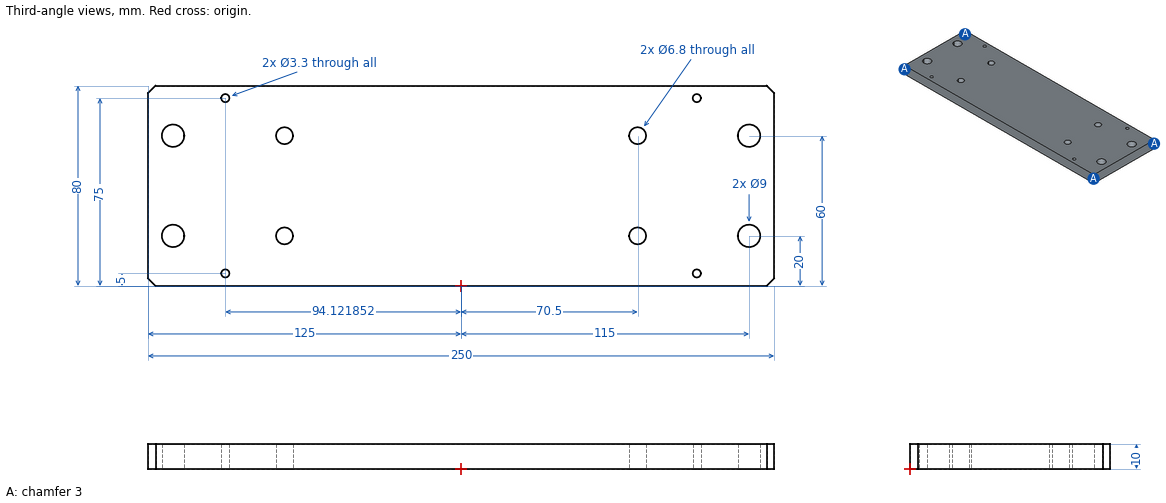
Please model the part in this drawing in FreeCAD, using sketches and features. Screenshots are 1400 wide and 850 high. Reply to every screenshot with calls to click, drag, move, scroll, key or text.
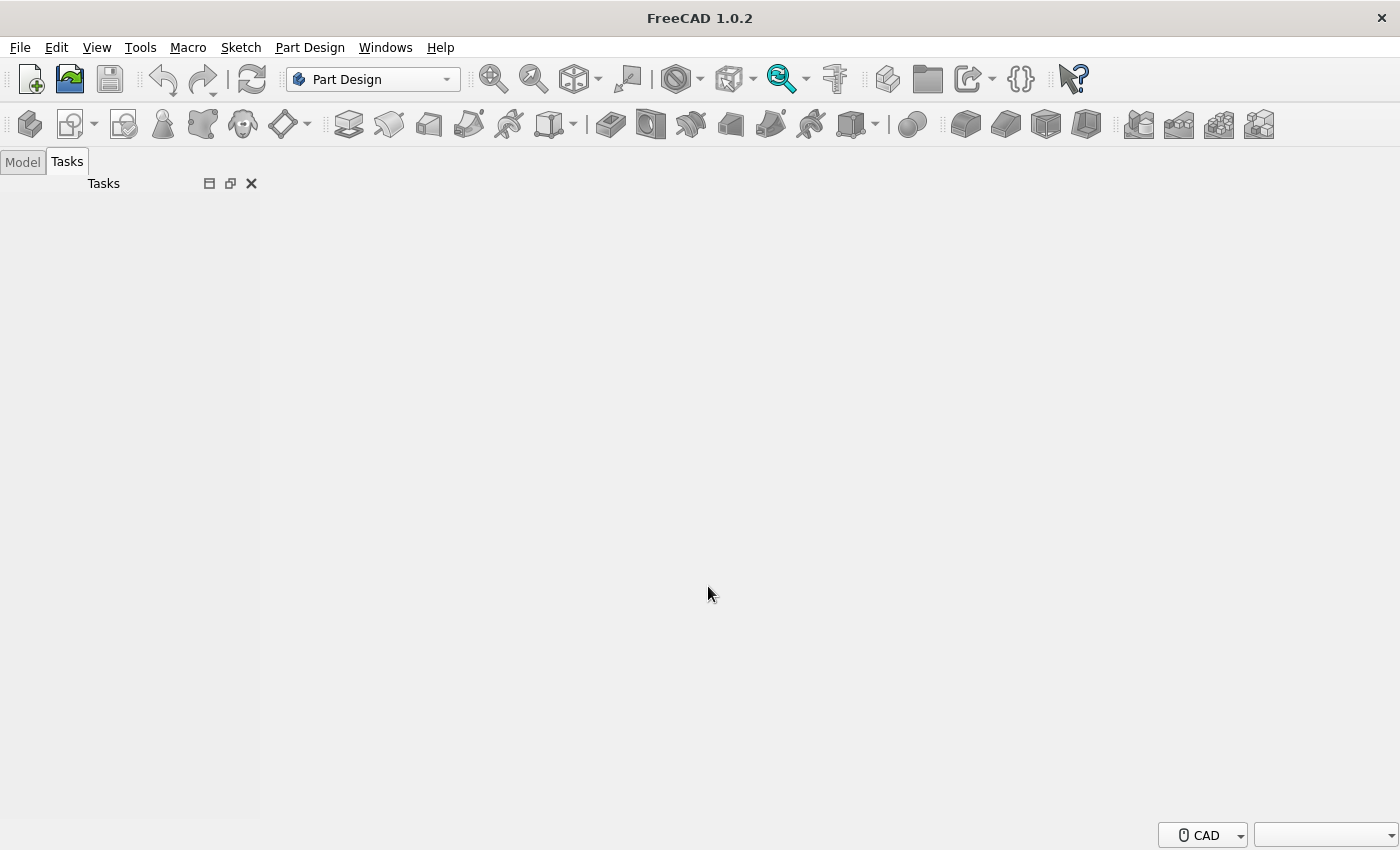
click(30, 80)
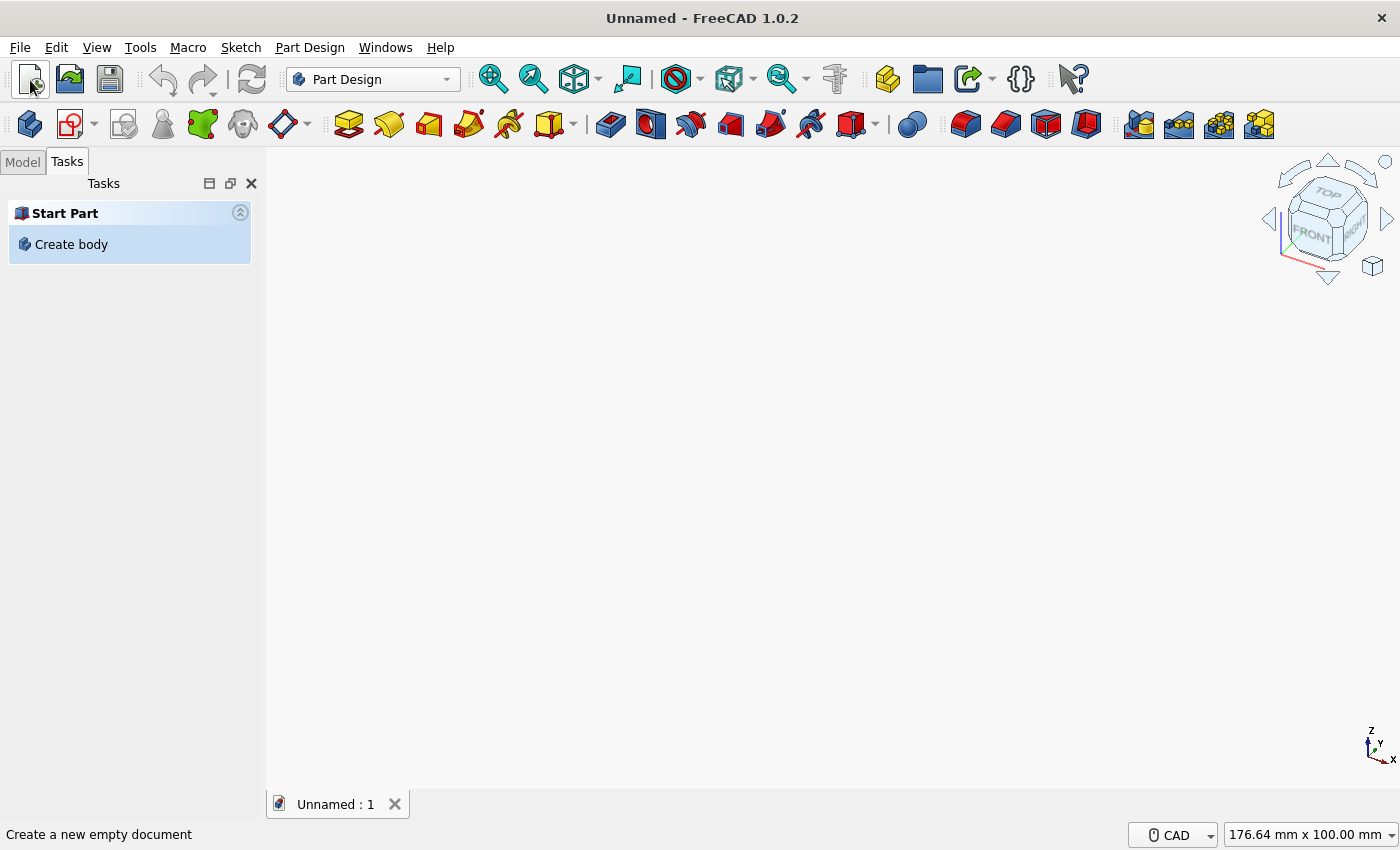
click(70, 124)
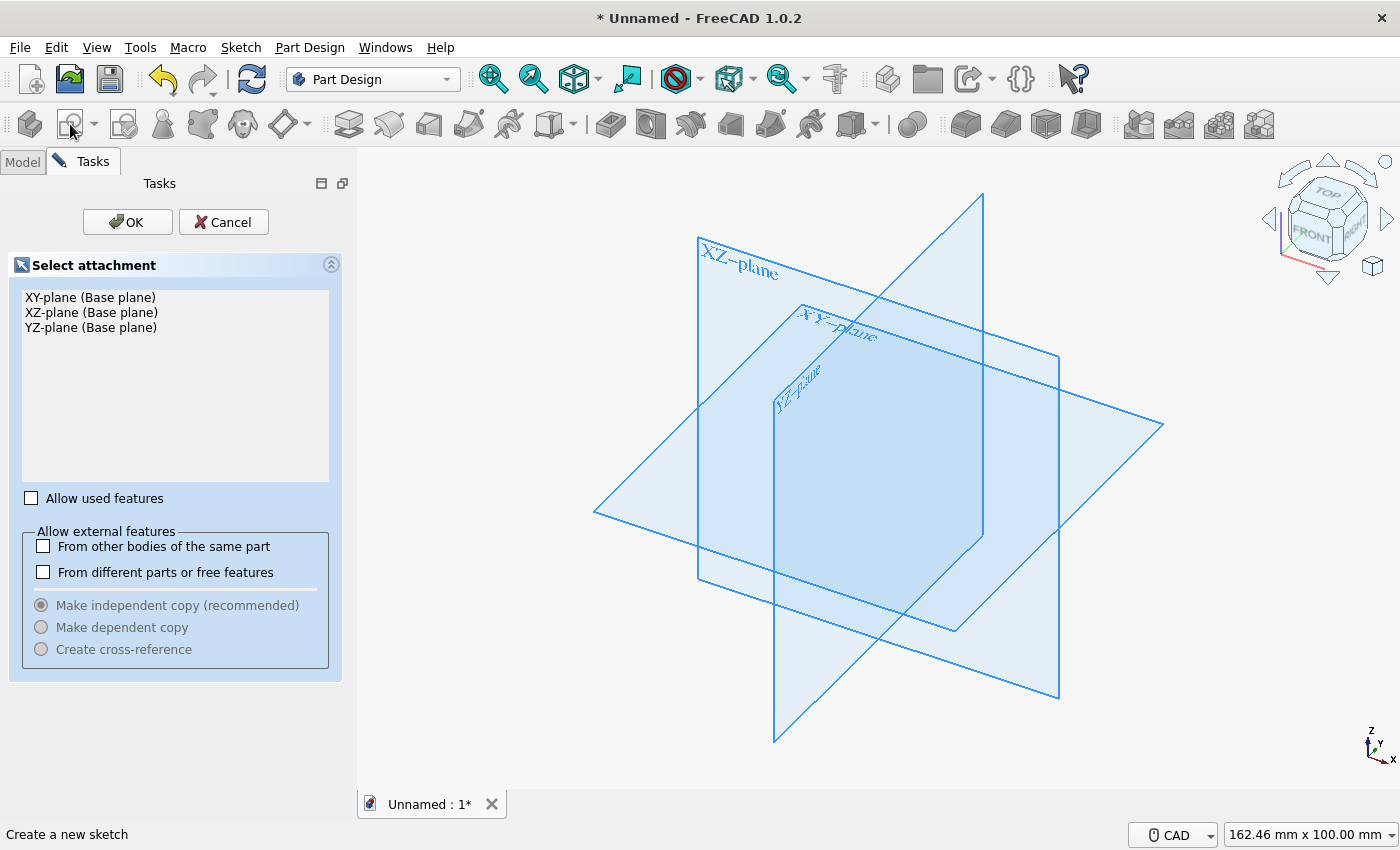
click(82, 298)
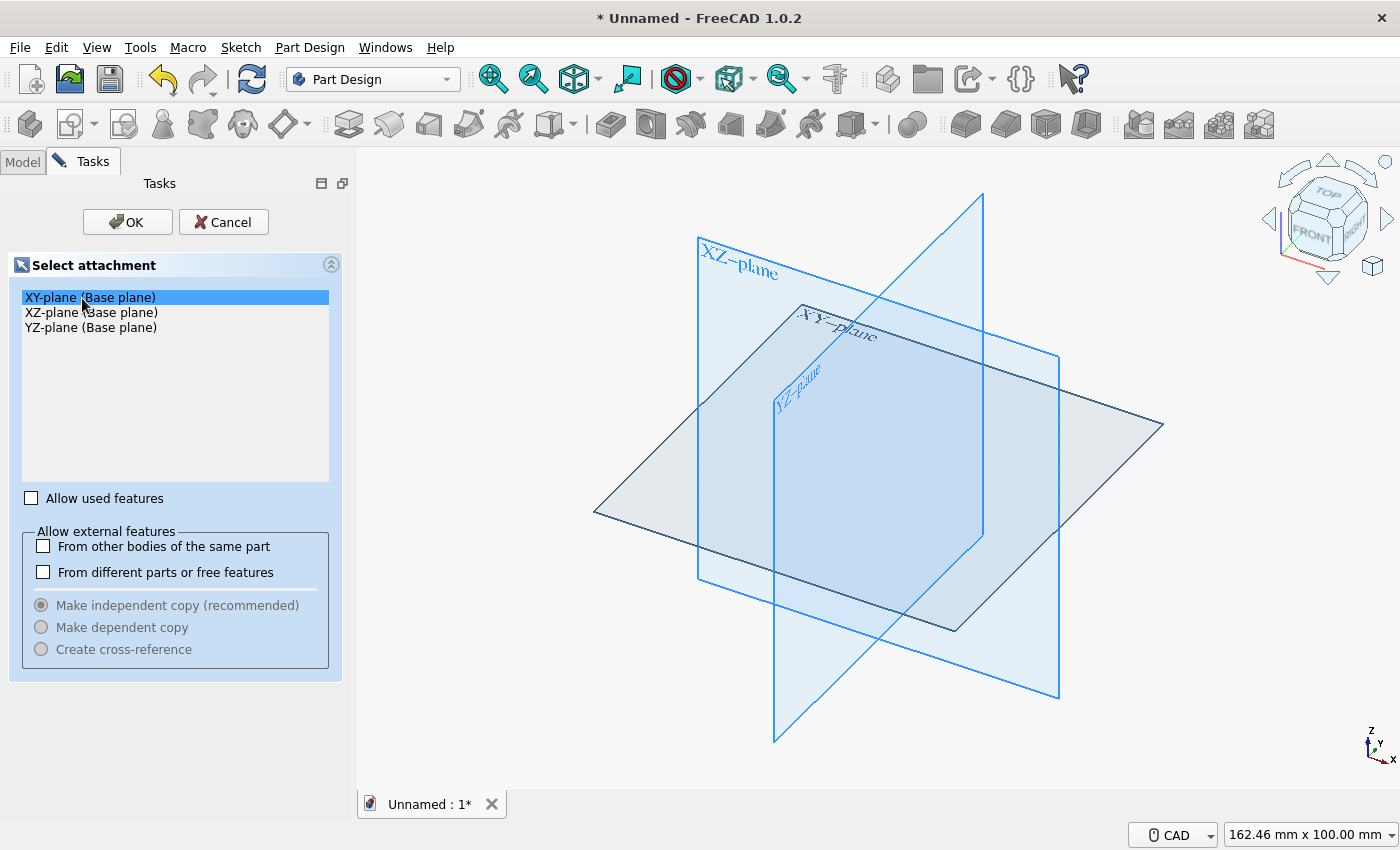
click(128, 222)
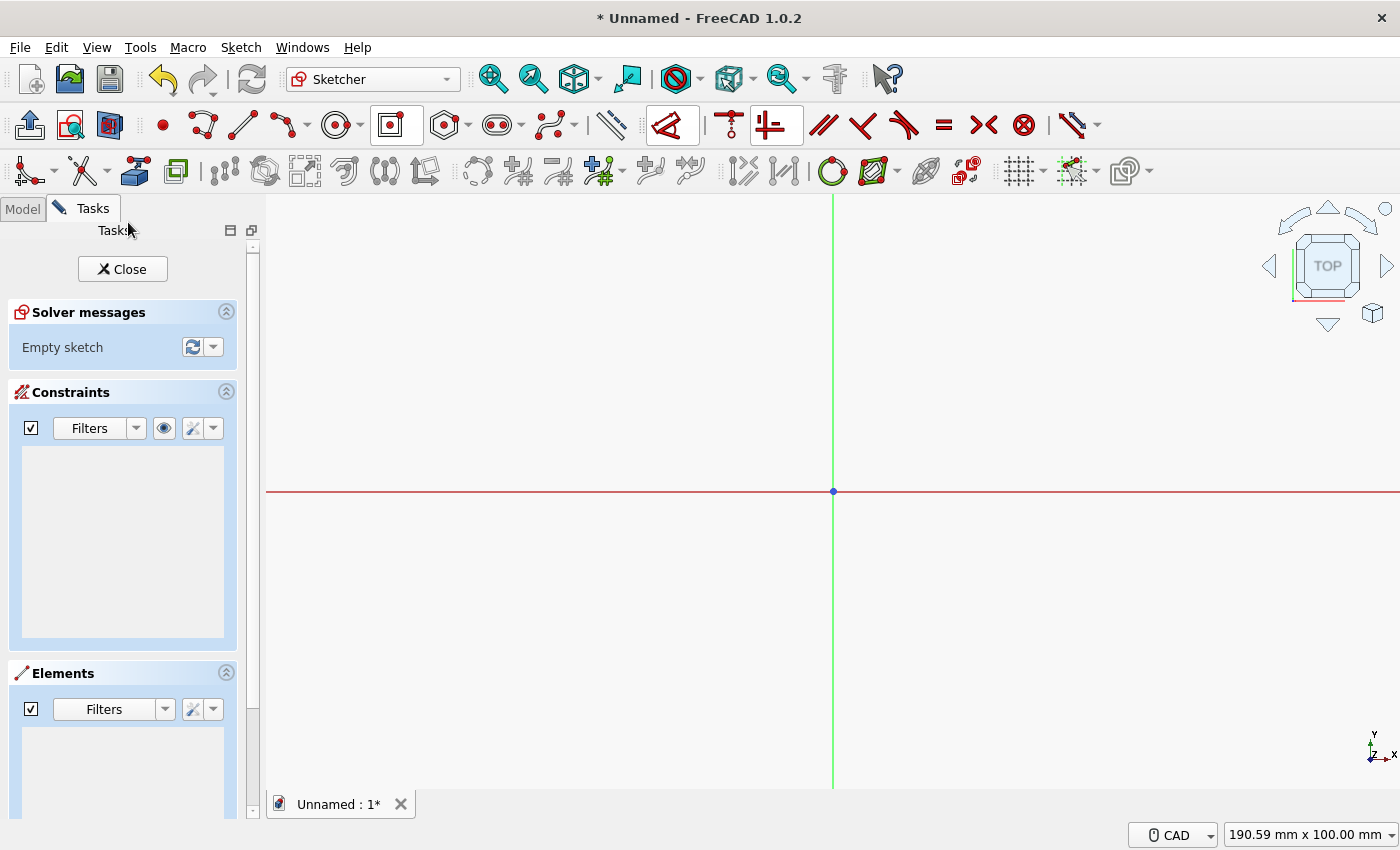
scroll(709, 686, down, 4)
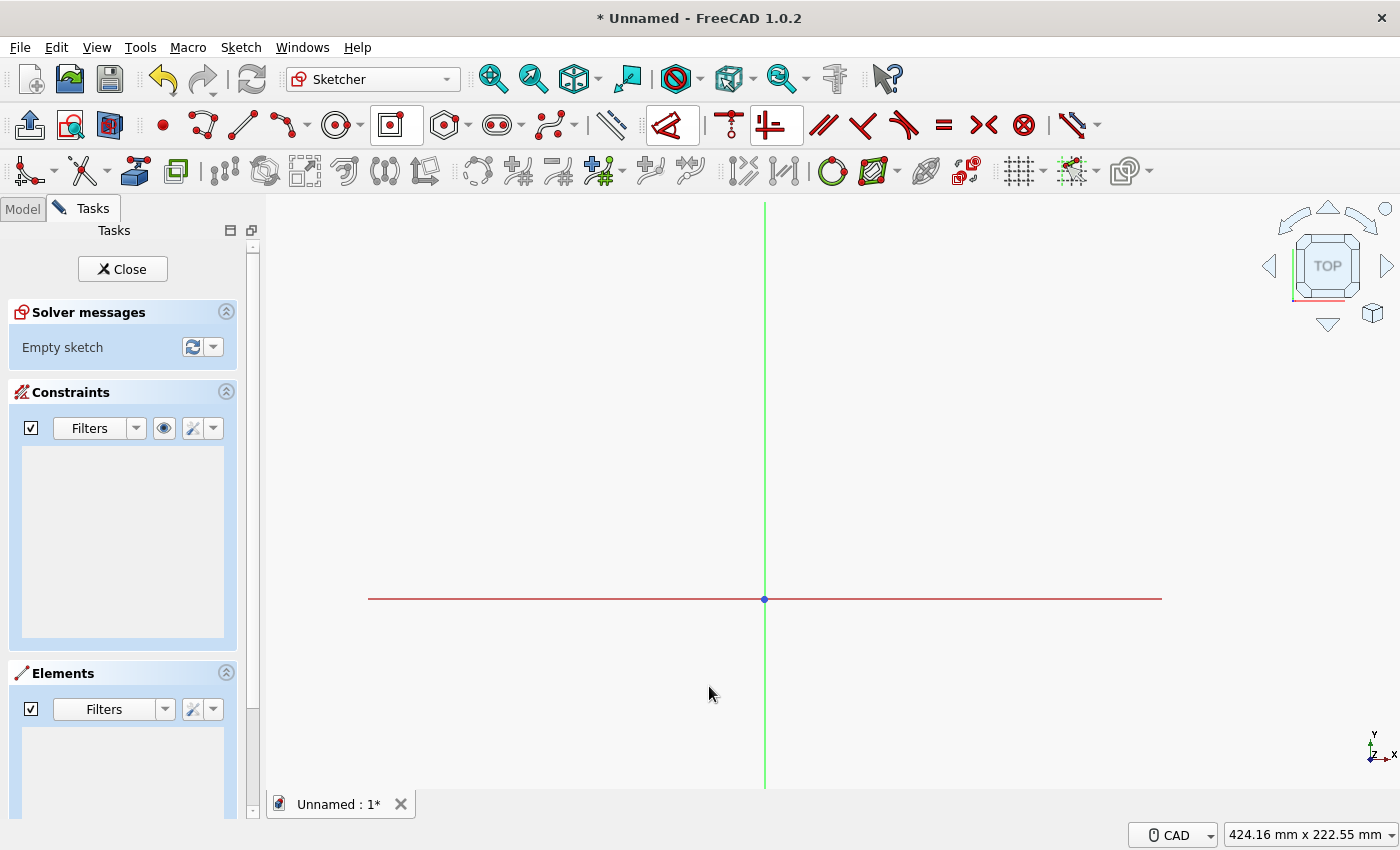
key(g)
key(r)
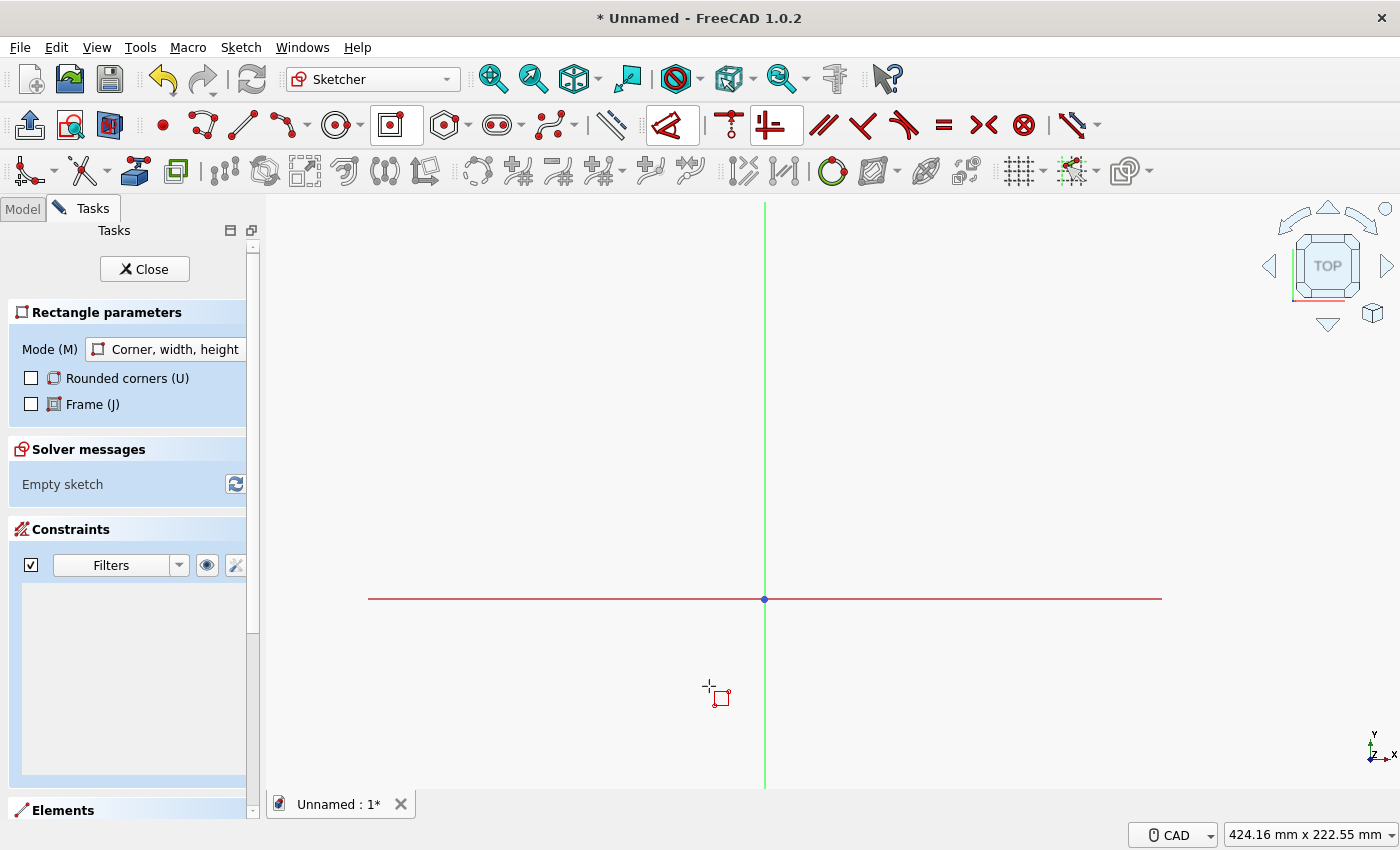
click(431, 385)
click(1099, 599)
key(Escape)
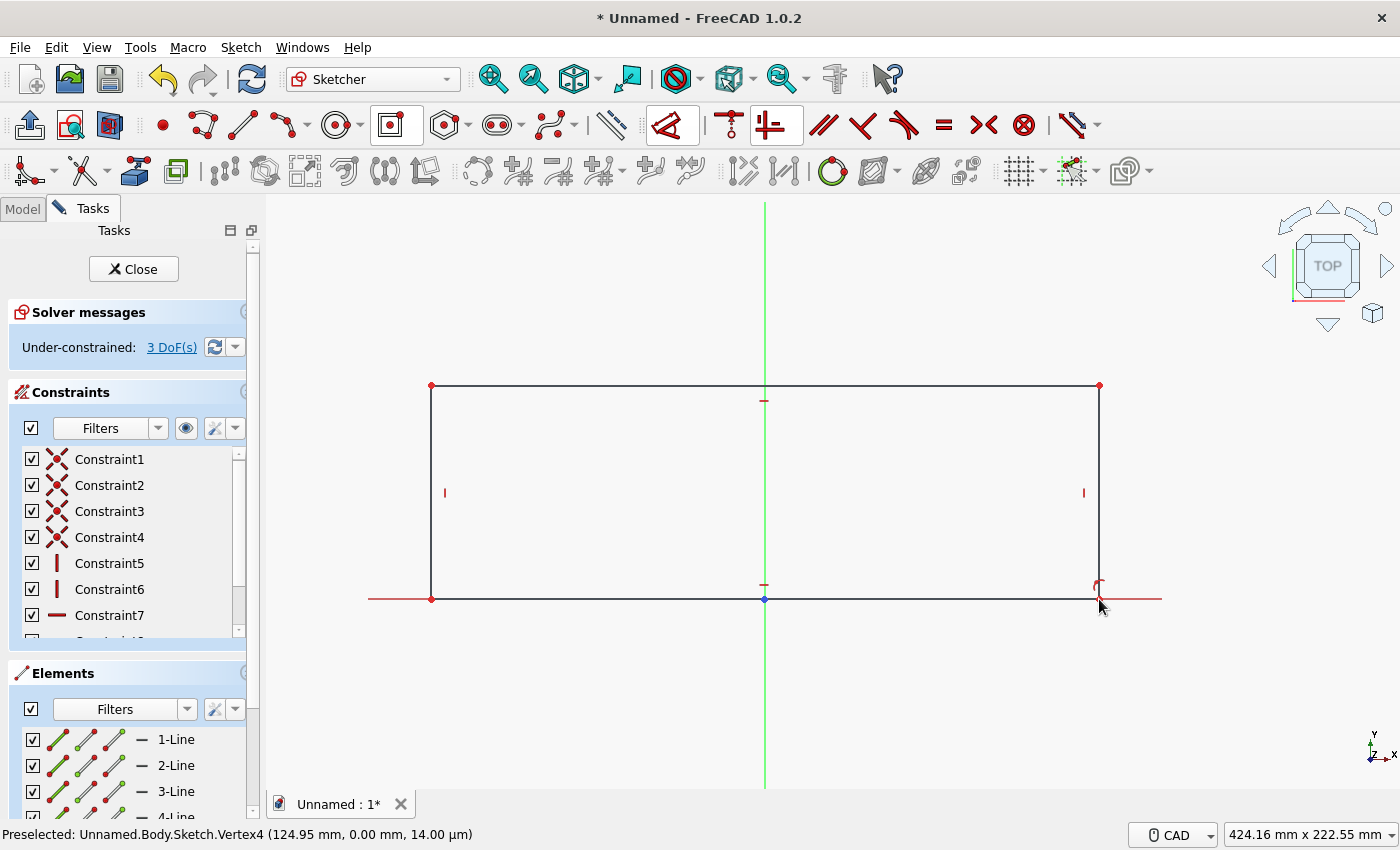
click(666, 126)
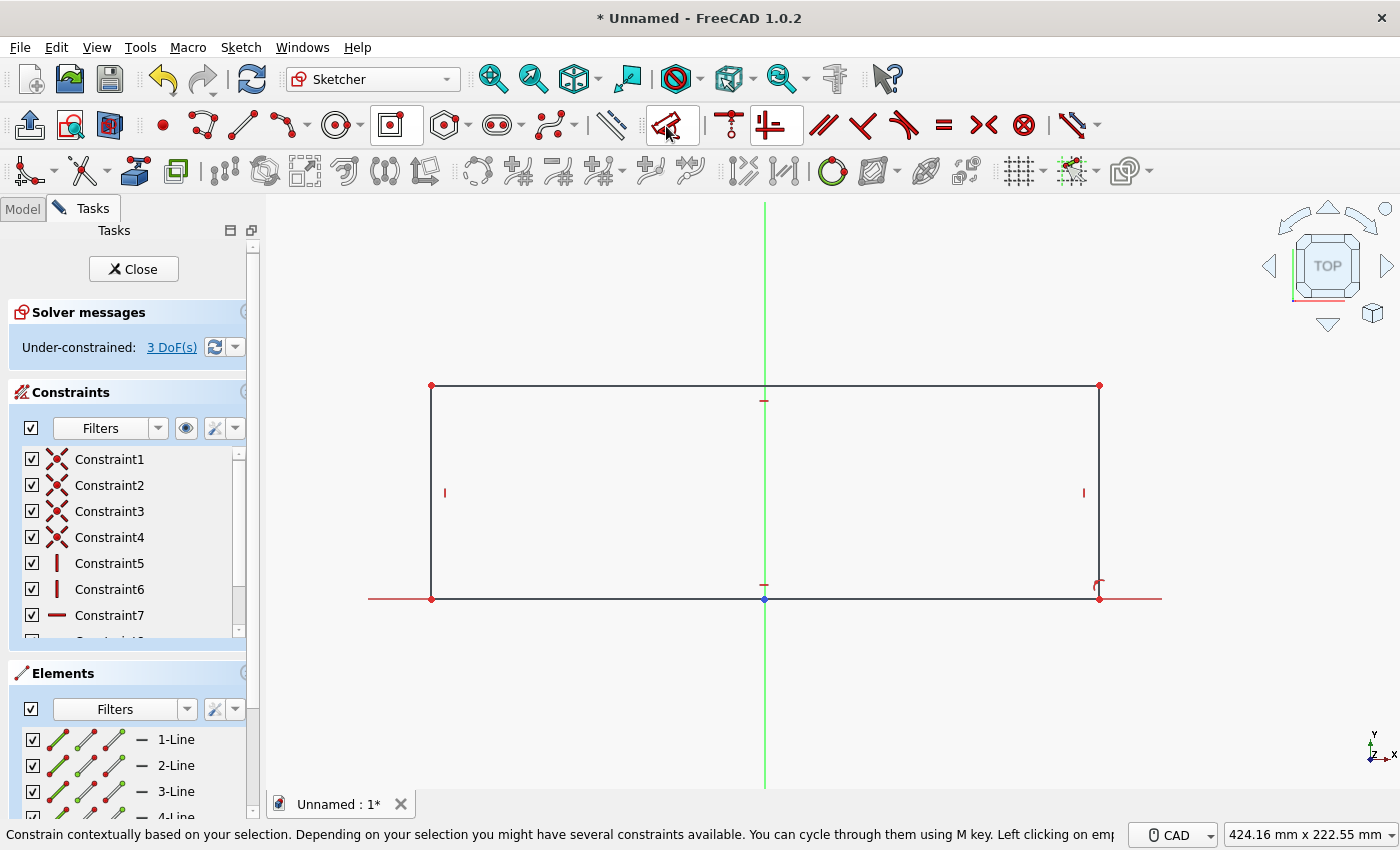
click(431, 450)
click(397, 493)